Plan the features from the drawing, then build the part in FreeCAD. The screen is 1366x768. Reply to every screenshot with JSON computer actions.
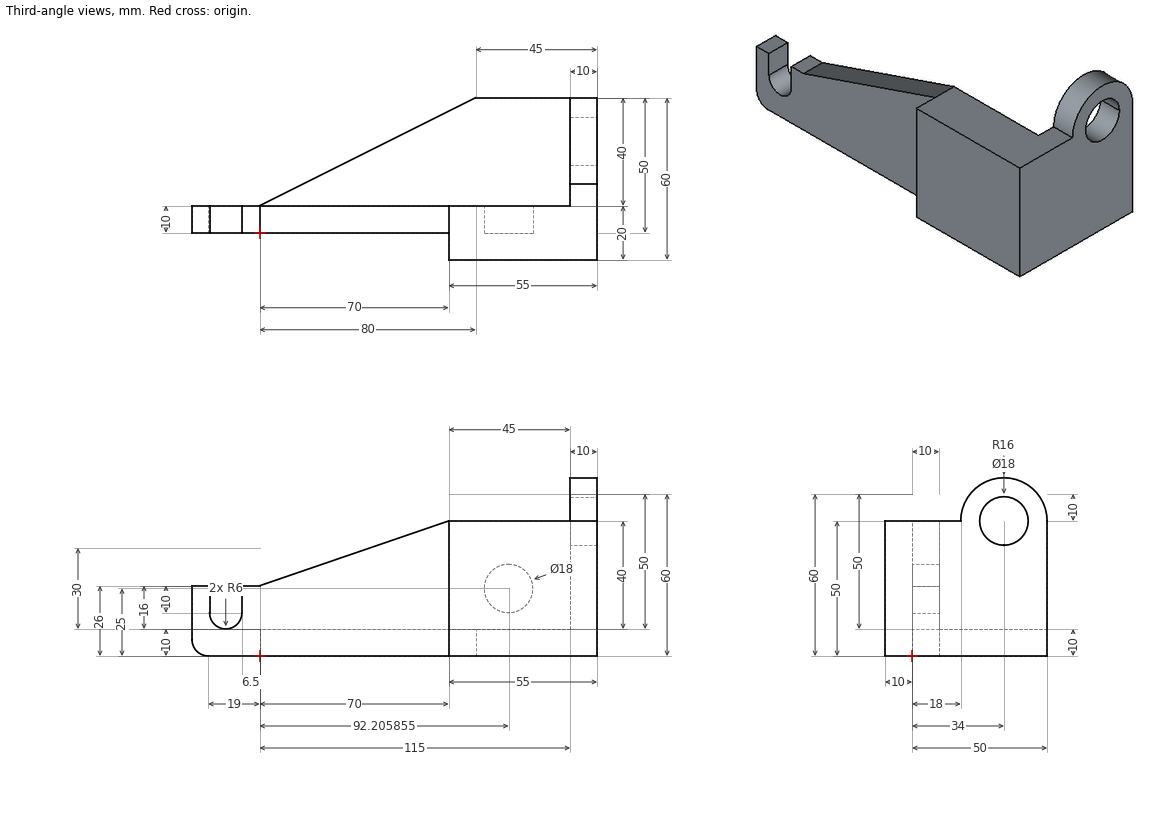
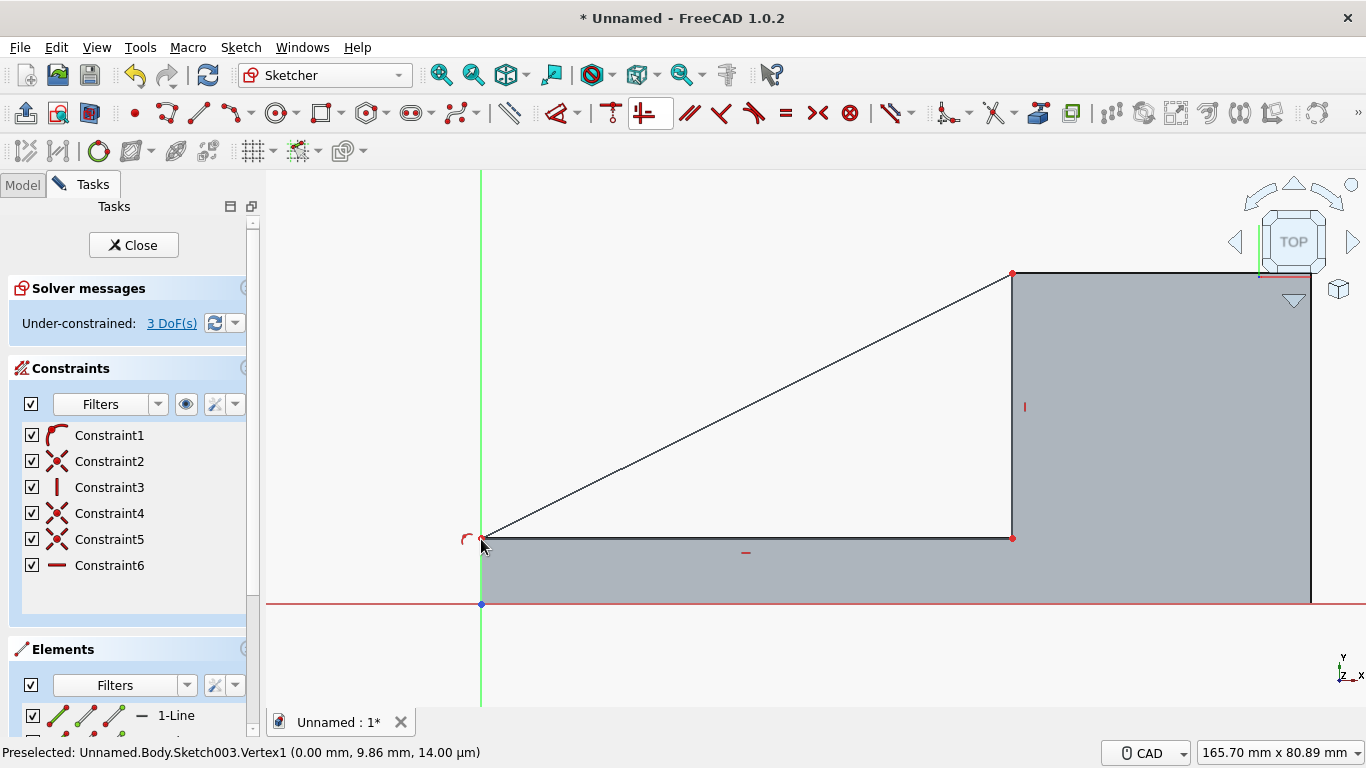
{"action": "left_click", "coordinate": [556, 114]}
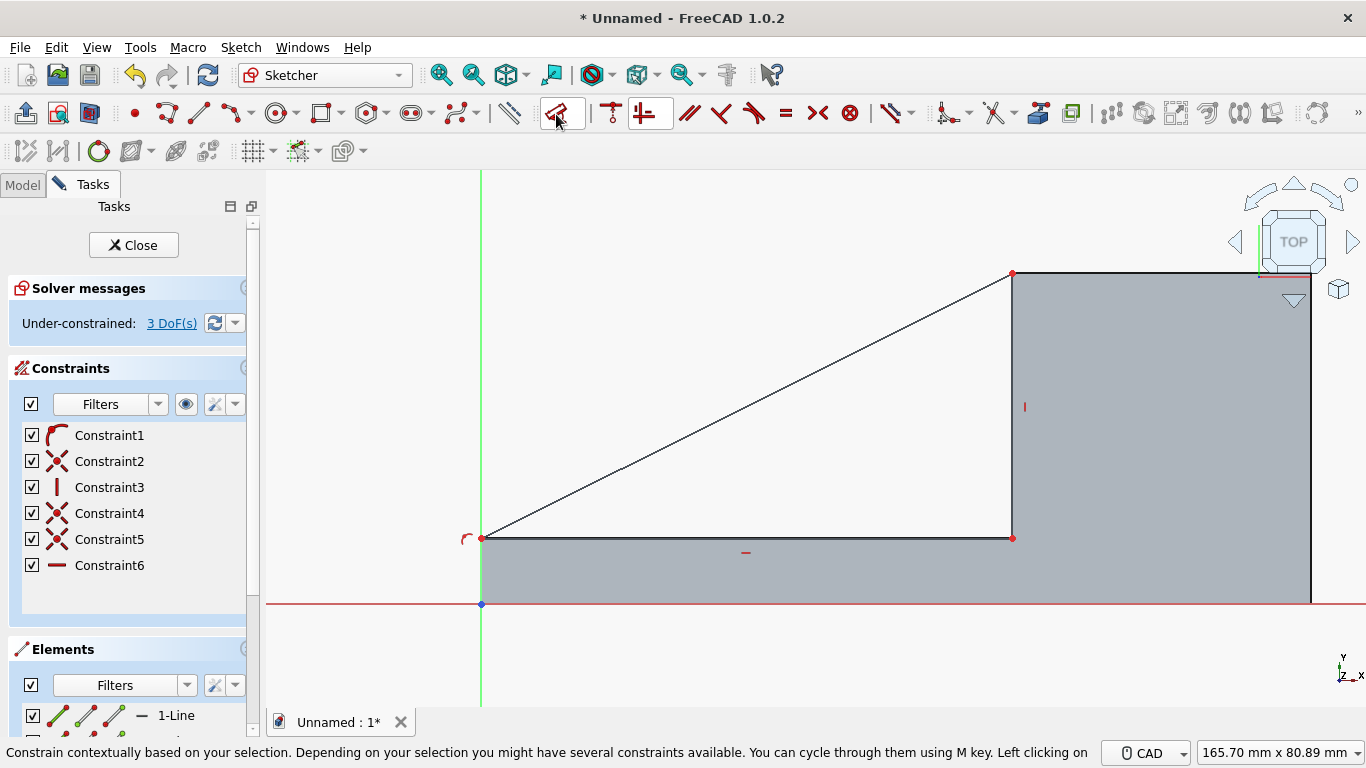
{"action": "left_click", "coordinate": [1012, 354]}
{"action": "left_click", "coordinate": [1046, 407]}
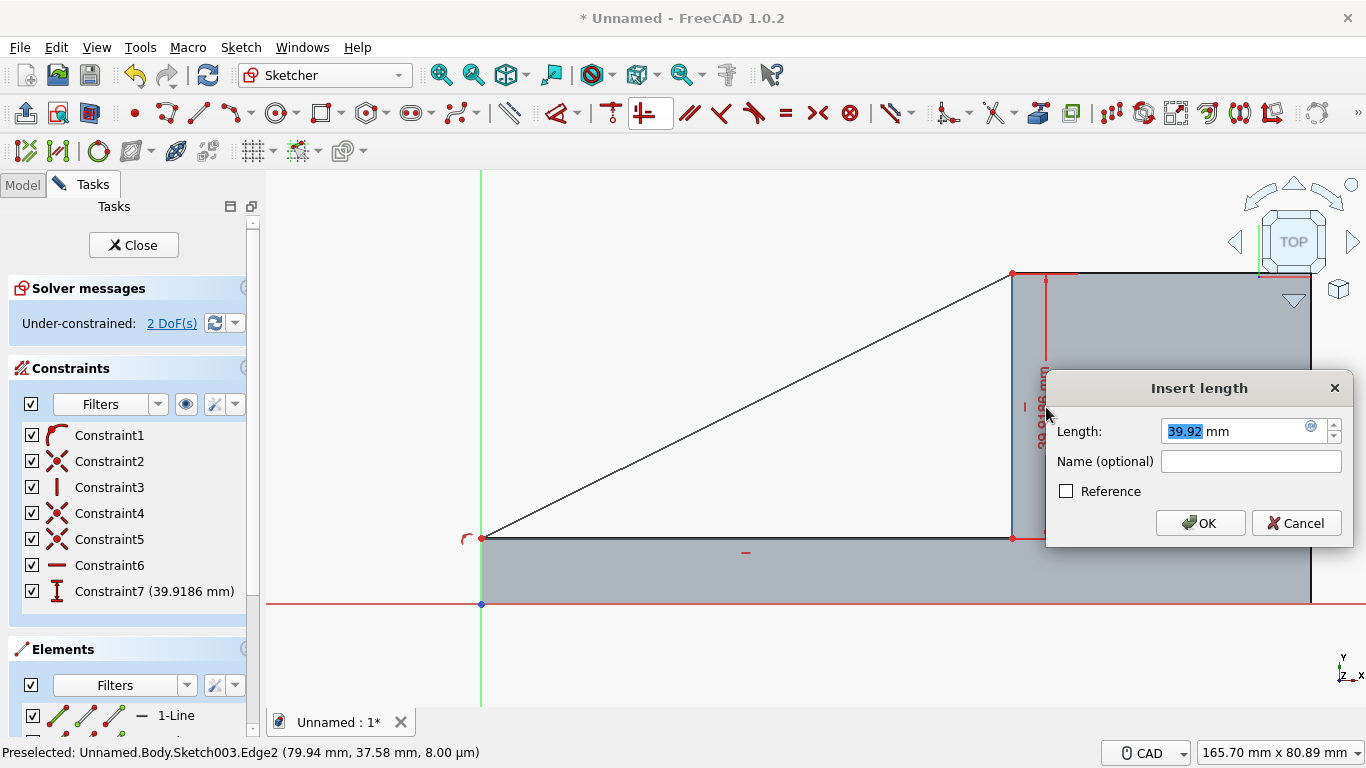
{"action": "type", "text": "40"}
{"action": "key", "text": "Return"}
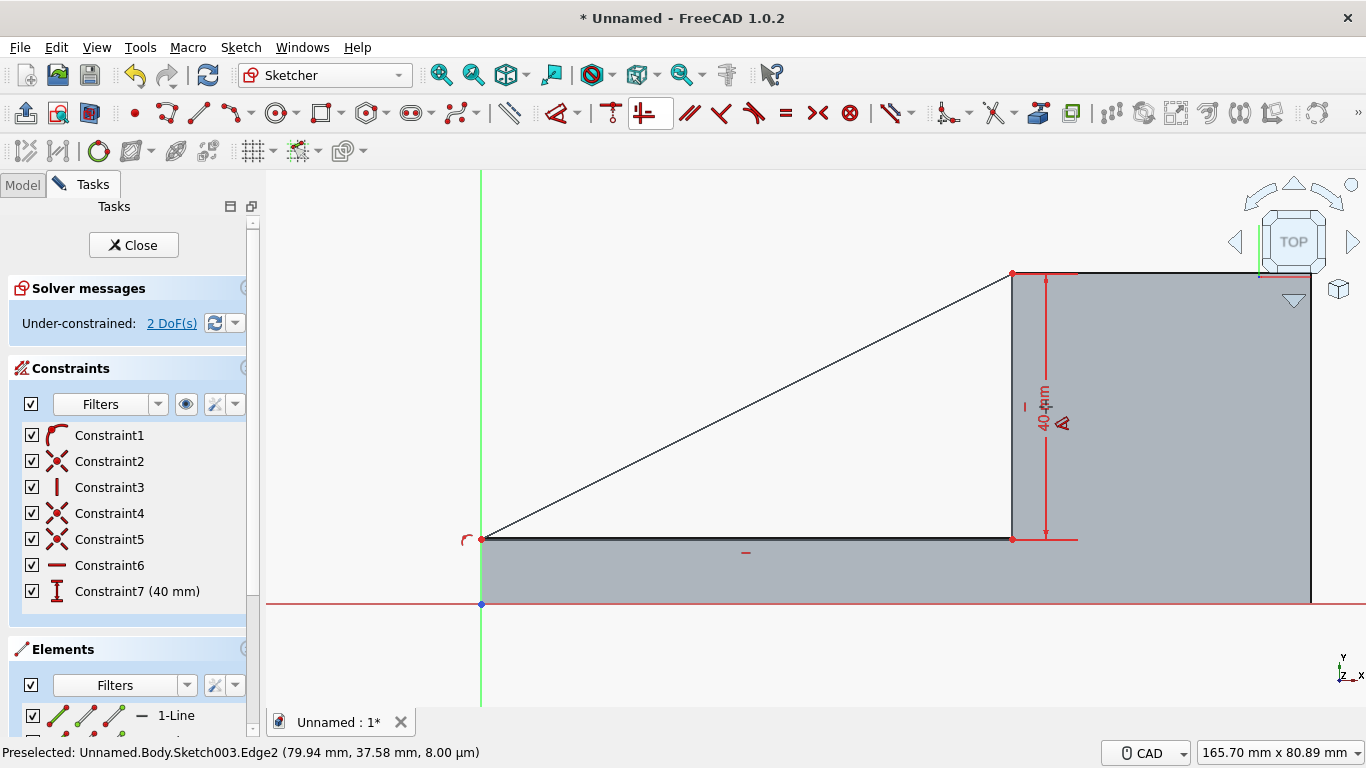
{"action": "left_click", "coordinate": [853, 540]}
{"action": "left_click", "coordinate": [747, 574]}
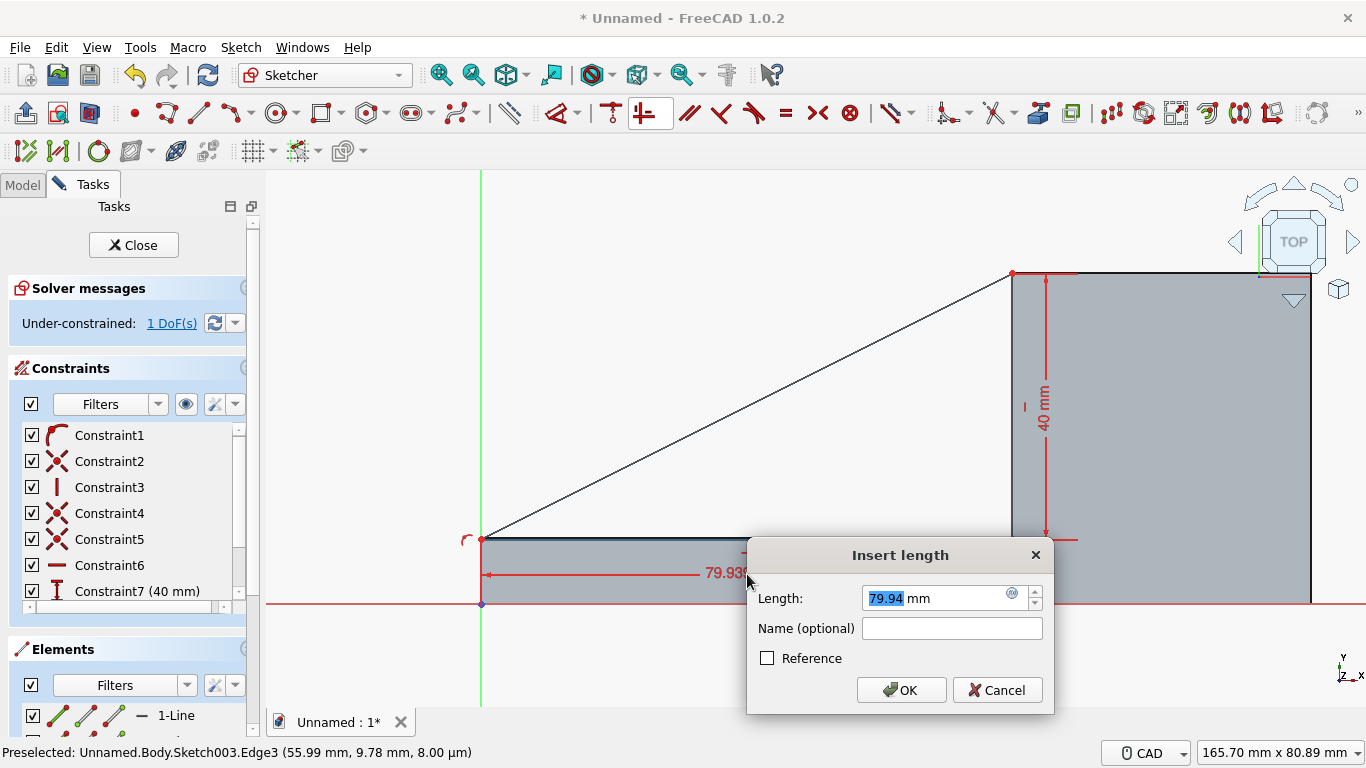
{"action": "type", "text": "80"}
{"action": "key", "text": "Return"}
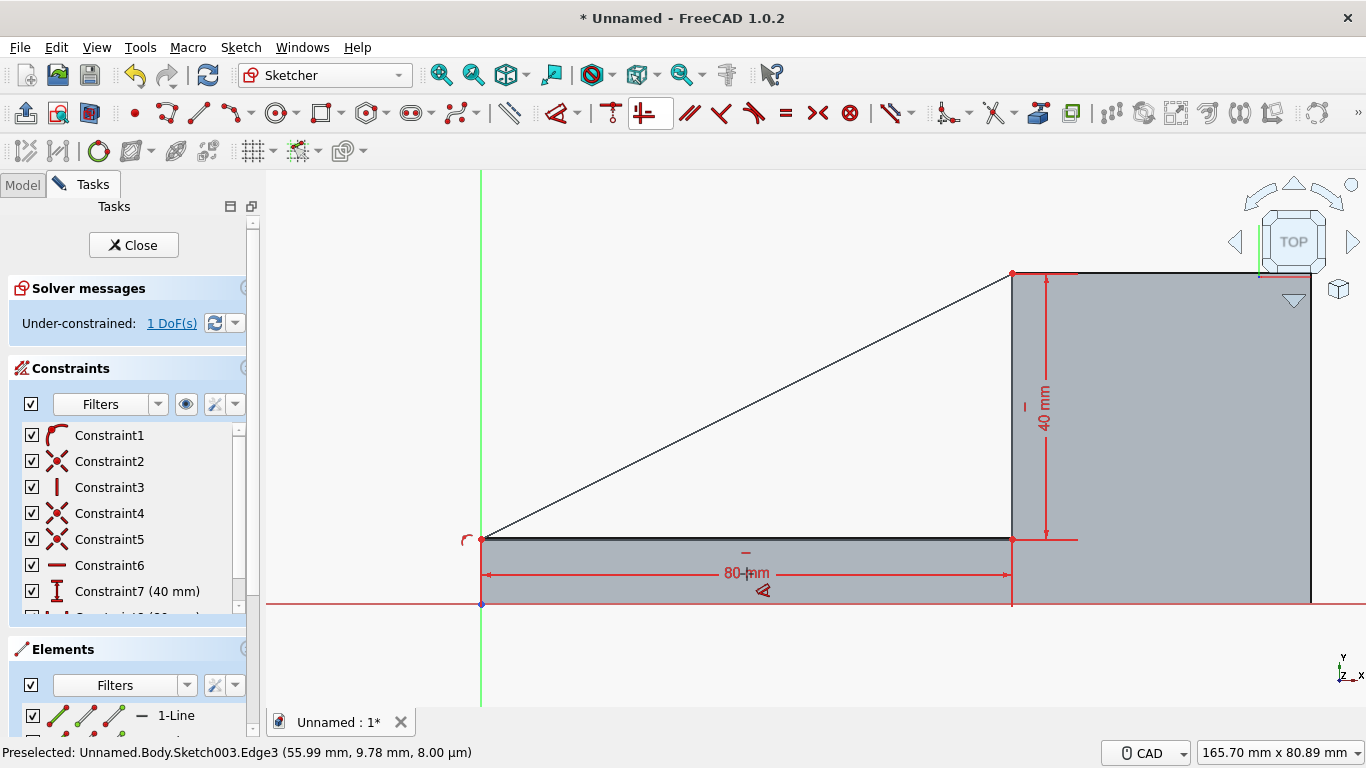
{"action": "left_click", "coordinate": [481, 540]}
{"action": "left_click", "coordinate": [447, 572]}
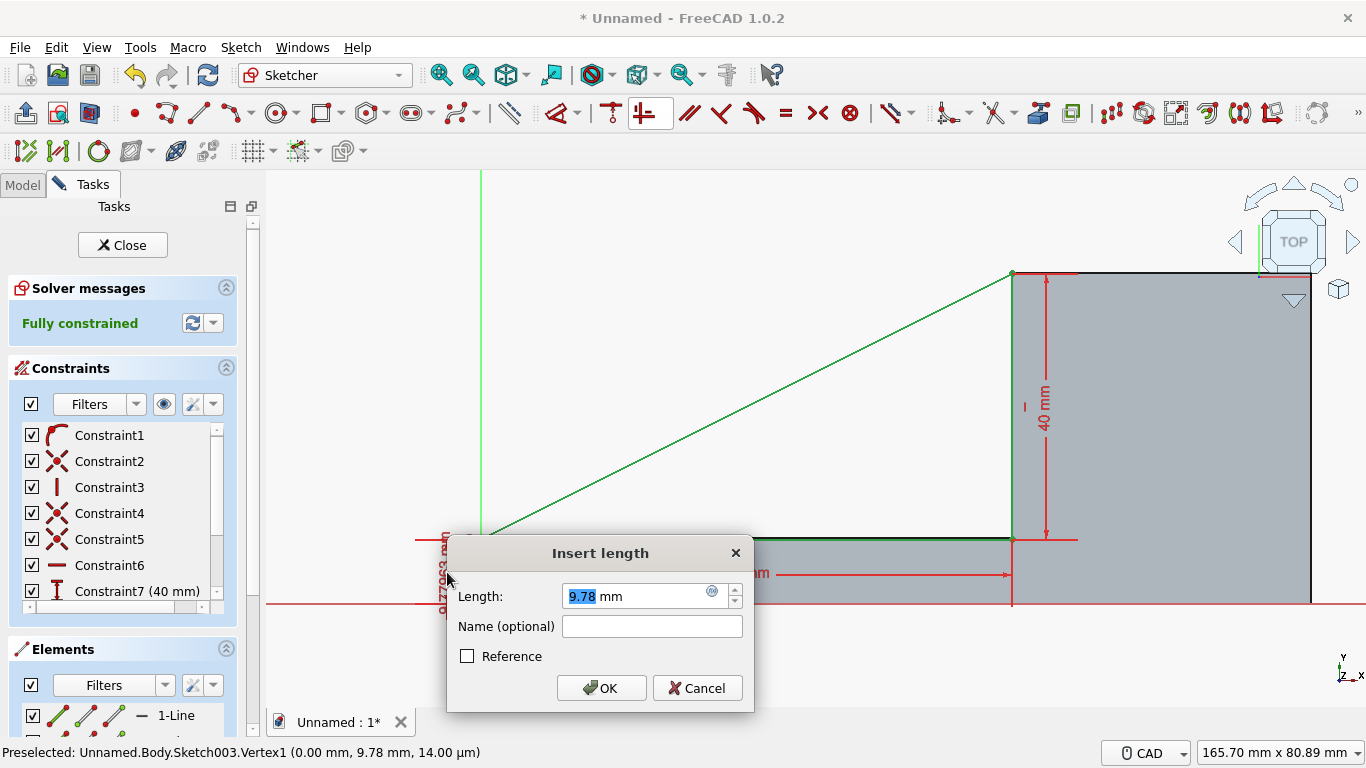
{"action": "type", "text": "10"}
{"action": "key", "text": "Return"}
{"action": "key", "text": "Escape"}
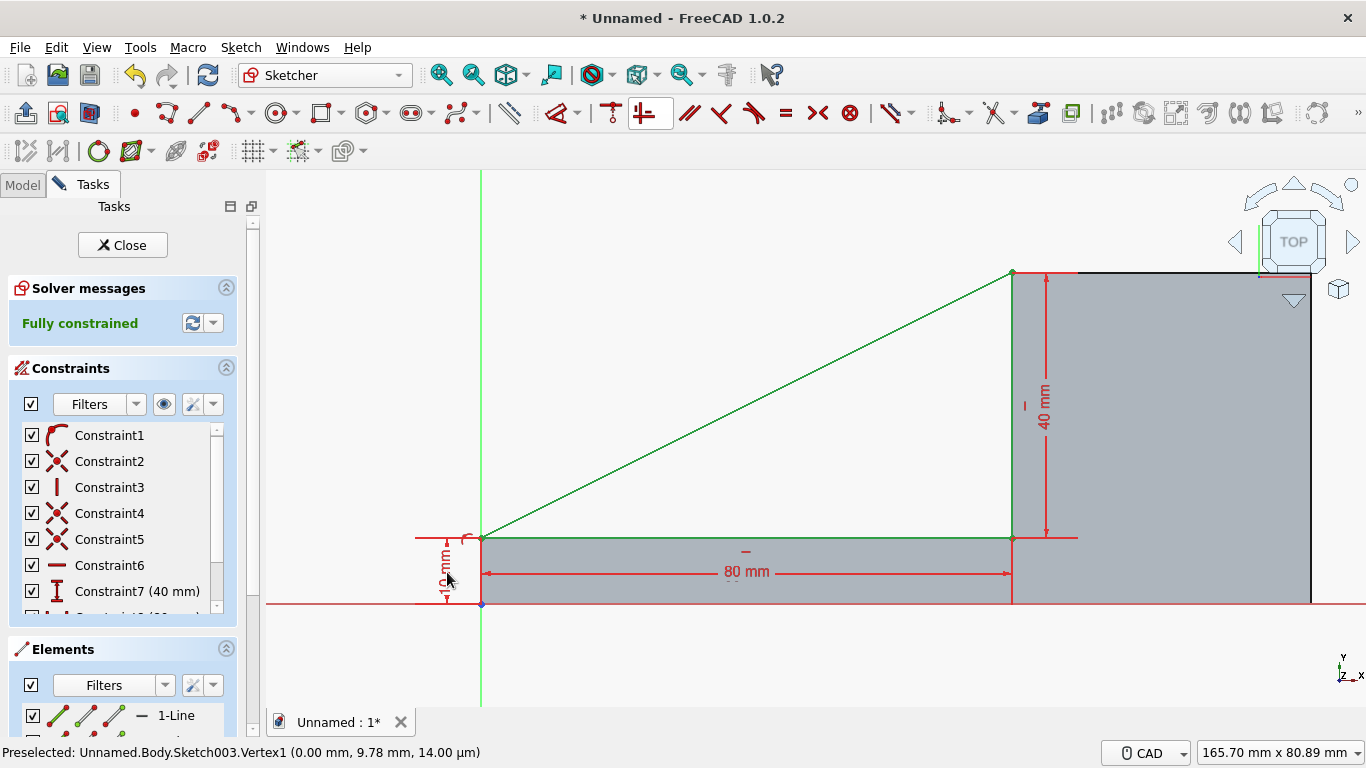
{"action": "left_click", "coordinate": [123, 245]}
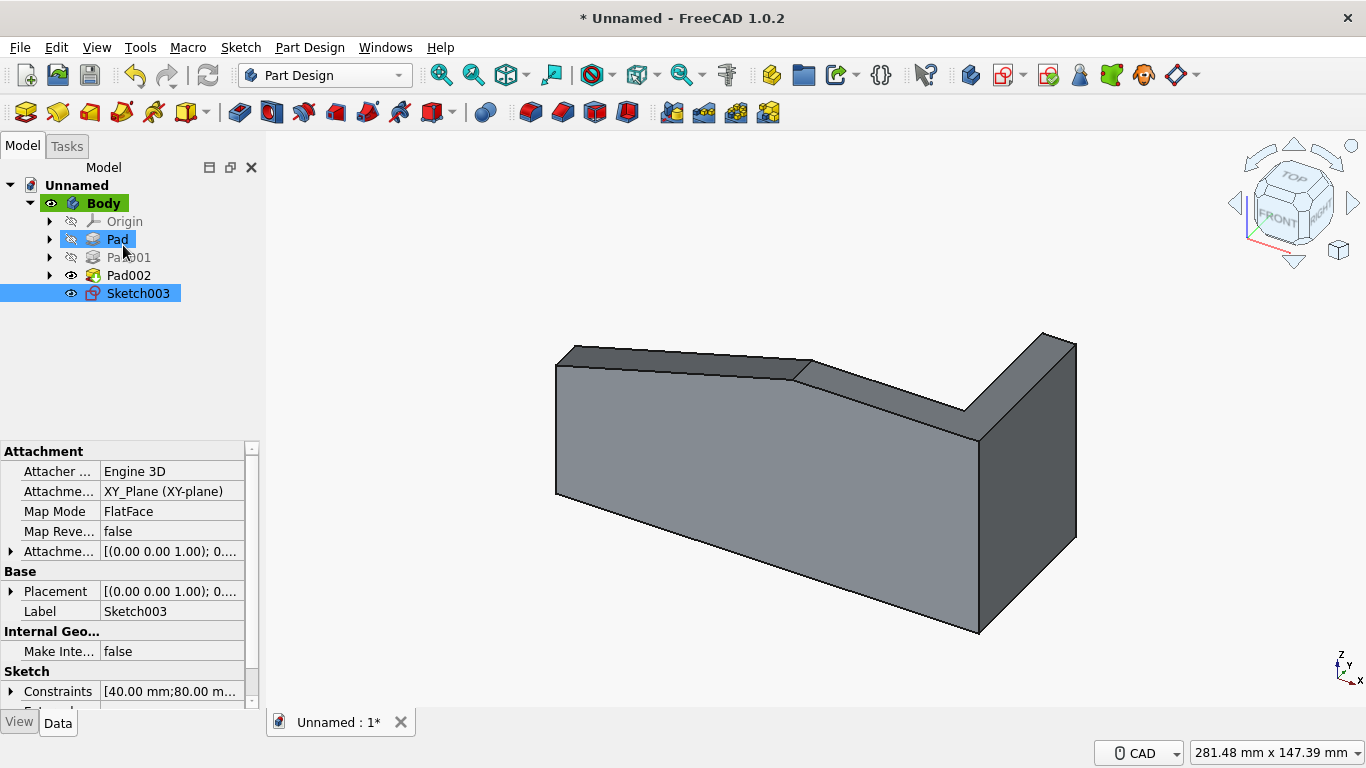
{"action": "left_click", "coordinate": [26, 112]}